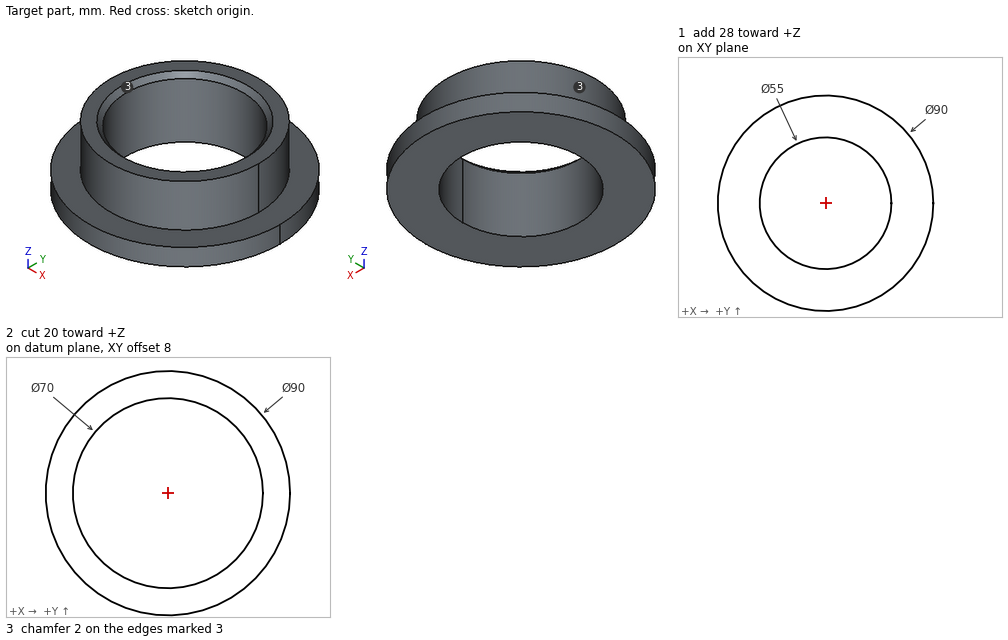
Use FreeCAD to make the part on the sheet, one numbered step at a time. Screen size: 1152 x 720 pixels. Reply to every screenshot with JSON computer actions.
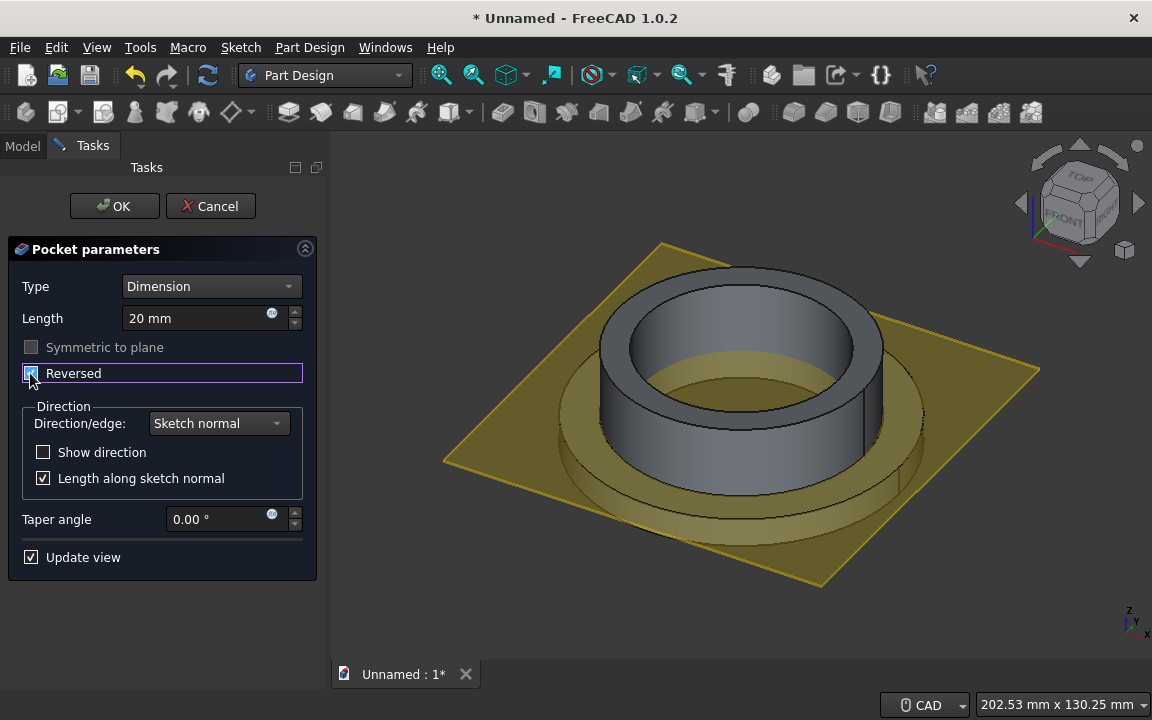
{"action": "left_click", "coordinate": [115, 206]}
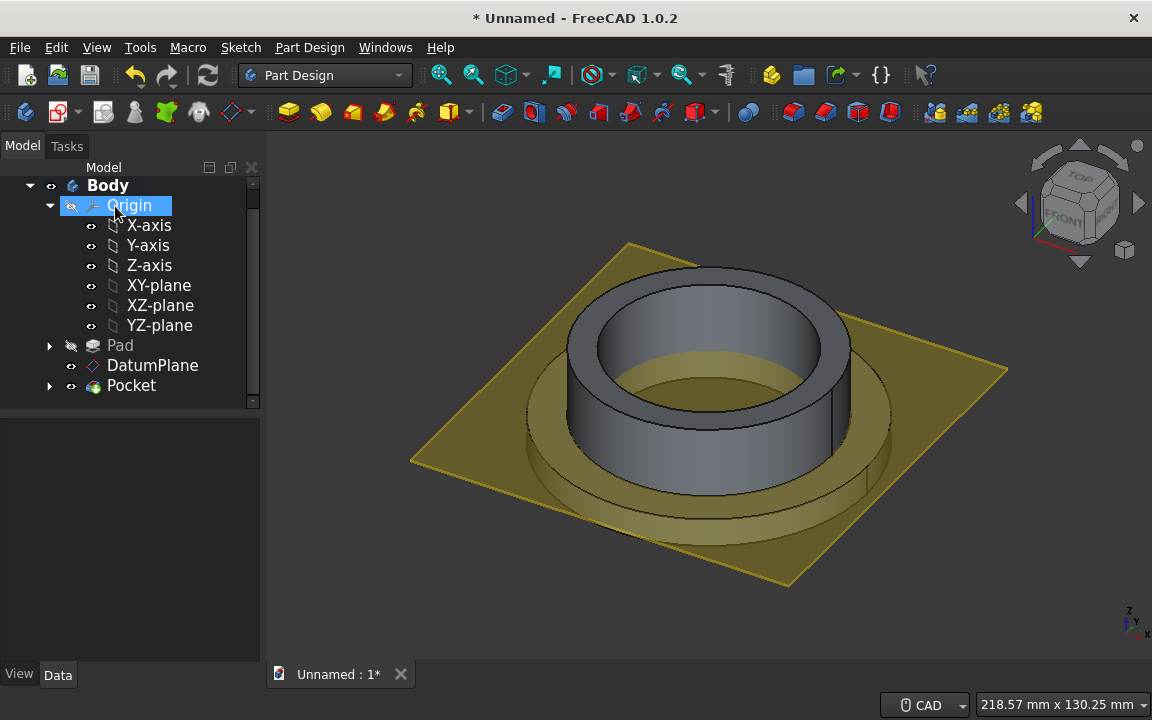
{"action": "left_click", "coordinate": [116, 366]}
{"action": "key", "text": "space"}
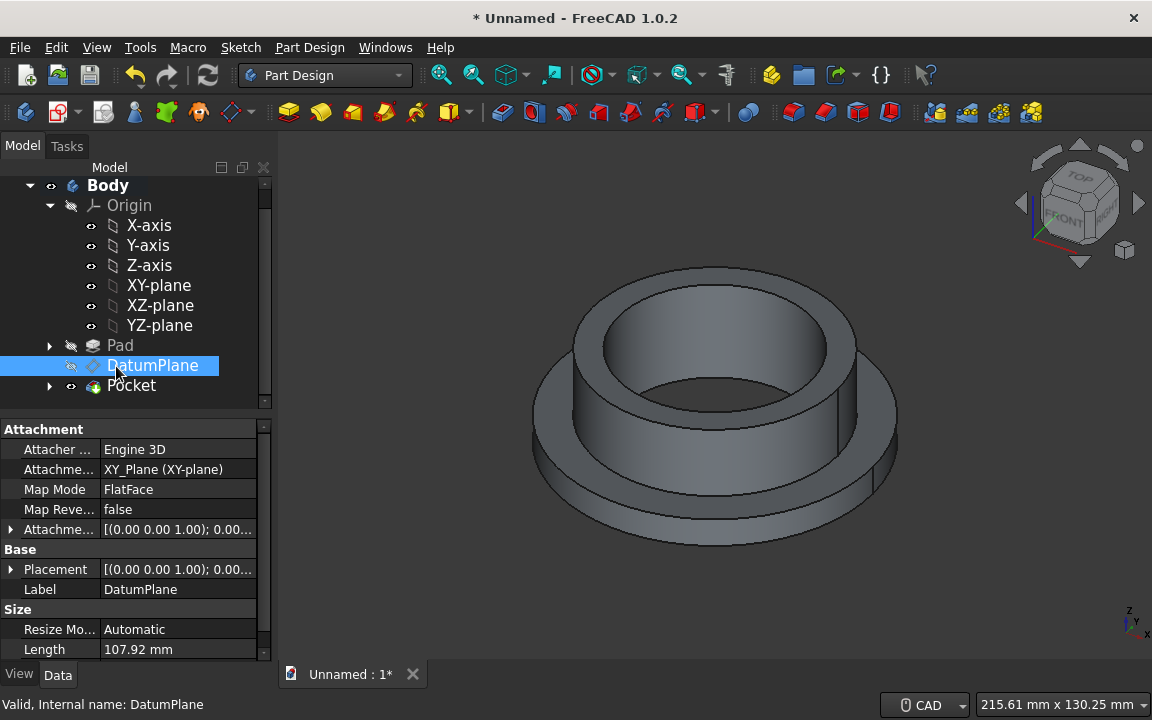
{"action": "left_click", "coordinate": [618, 316]}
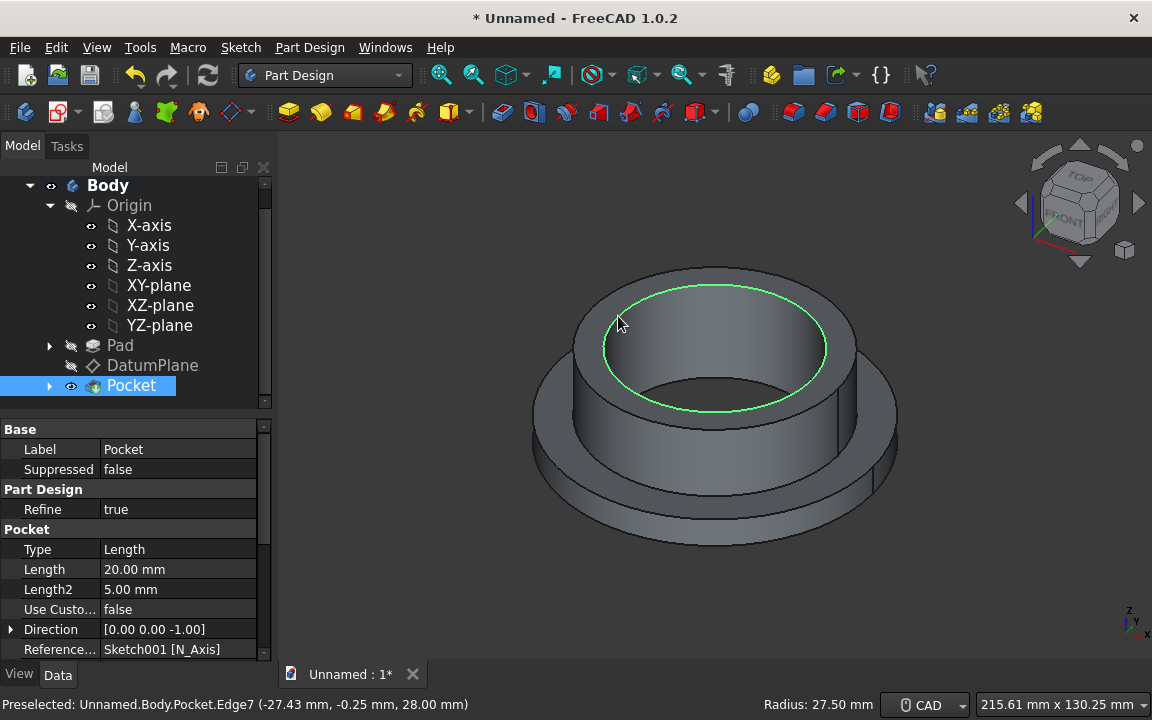
{"action": "left_click", "coordinate": [826, 112]}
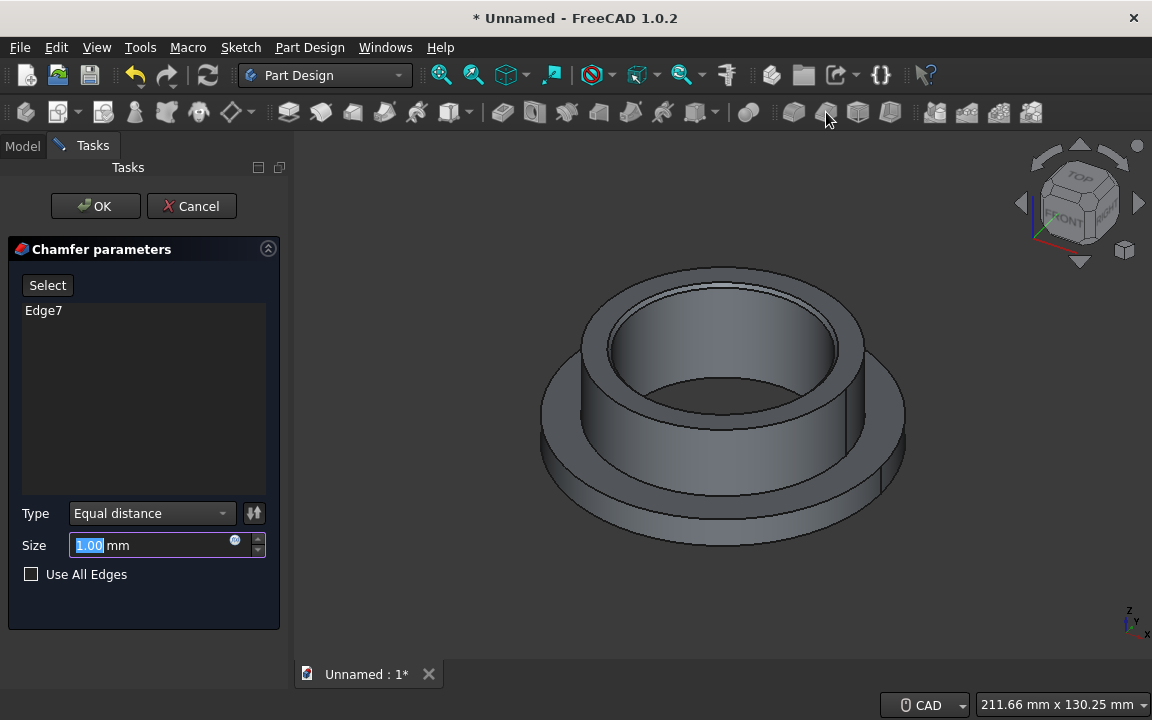
{"action": "type", "text": "2"}
{"action": "key", "text": "Tab"}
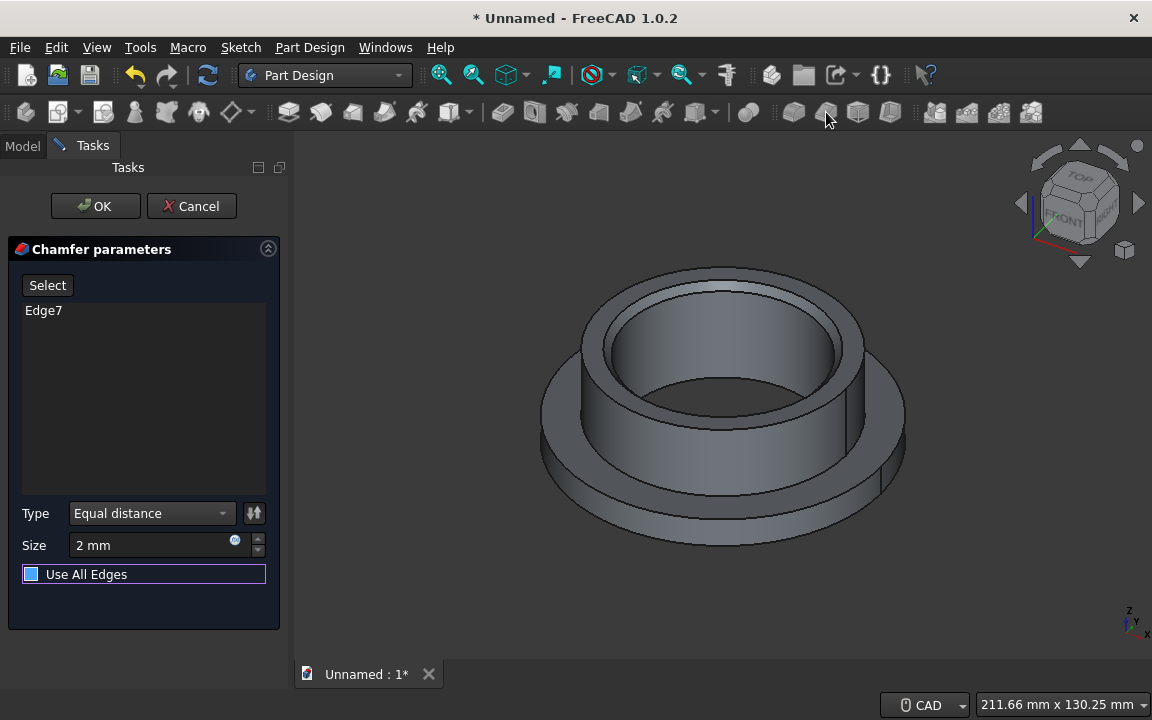
{"action": "left_click", "coordinate": [96, 206]}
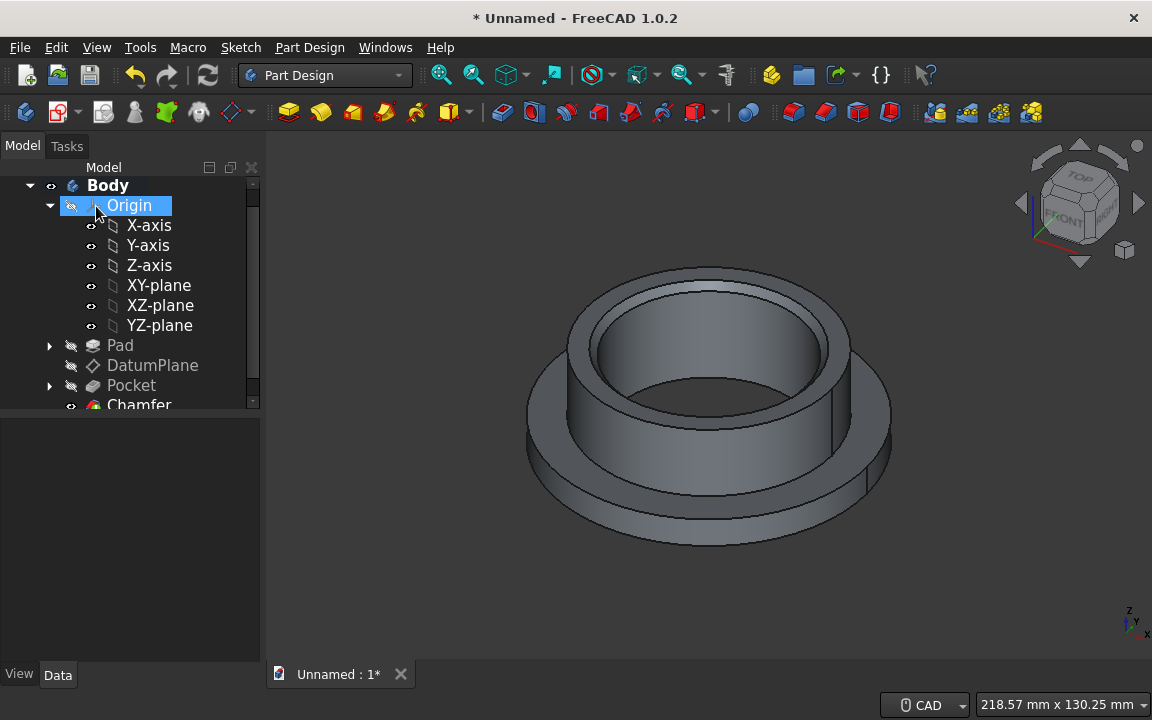
{"action": "key", "text": "0"}